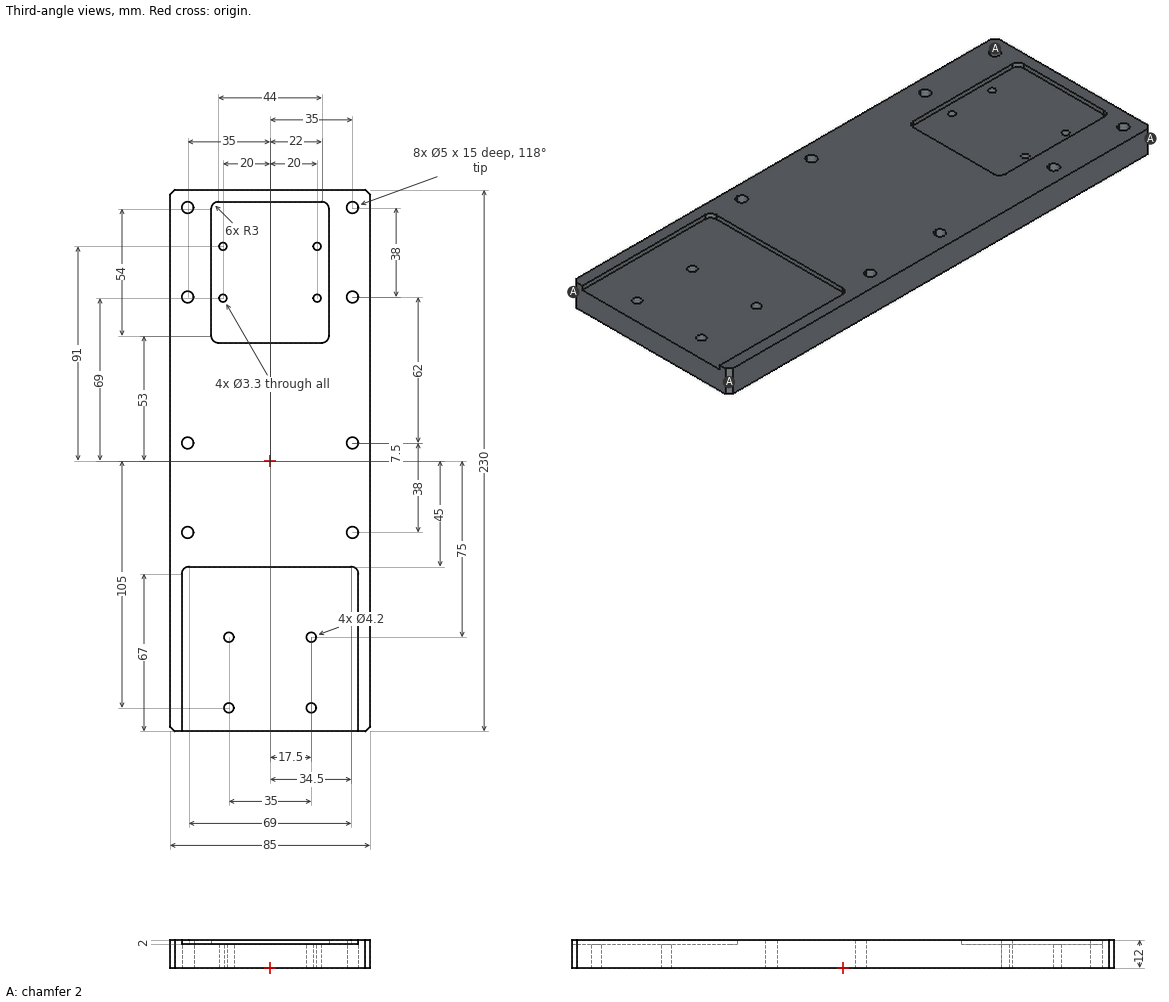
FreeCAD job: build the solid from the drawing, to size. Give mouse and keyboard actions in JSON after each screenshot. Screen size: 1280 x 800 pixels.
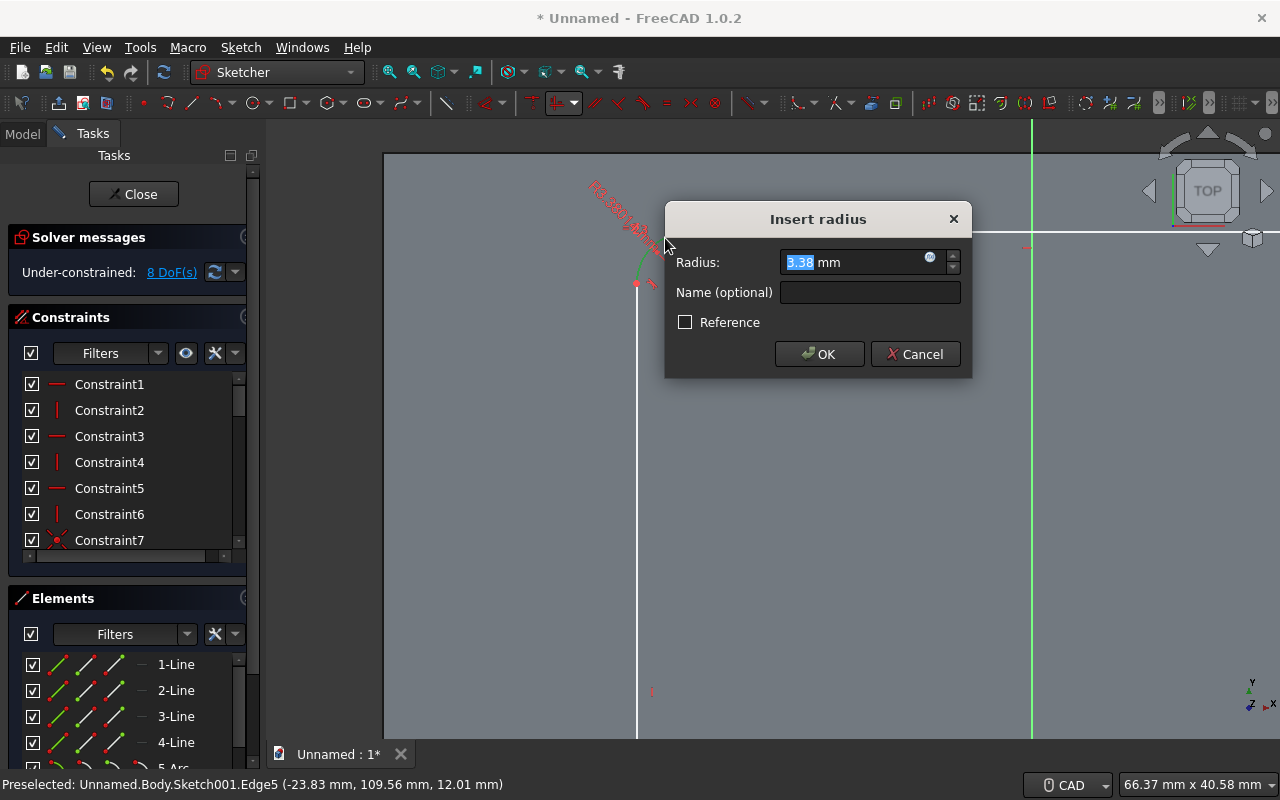
{"action": "type", "text": "3"}
{"action": "key", "text": "Return"}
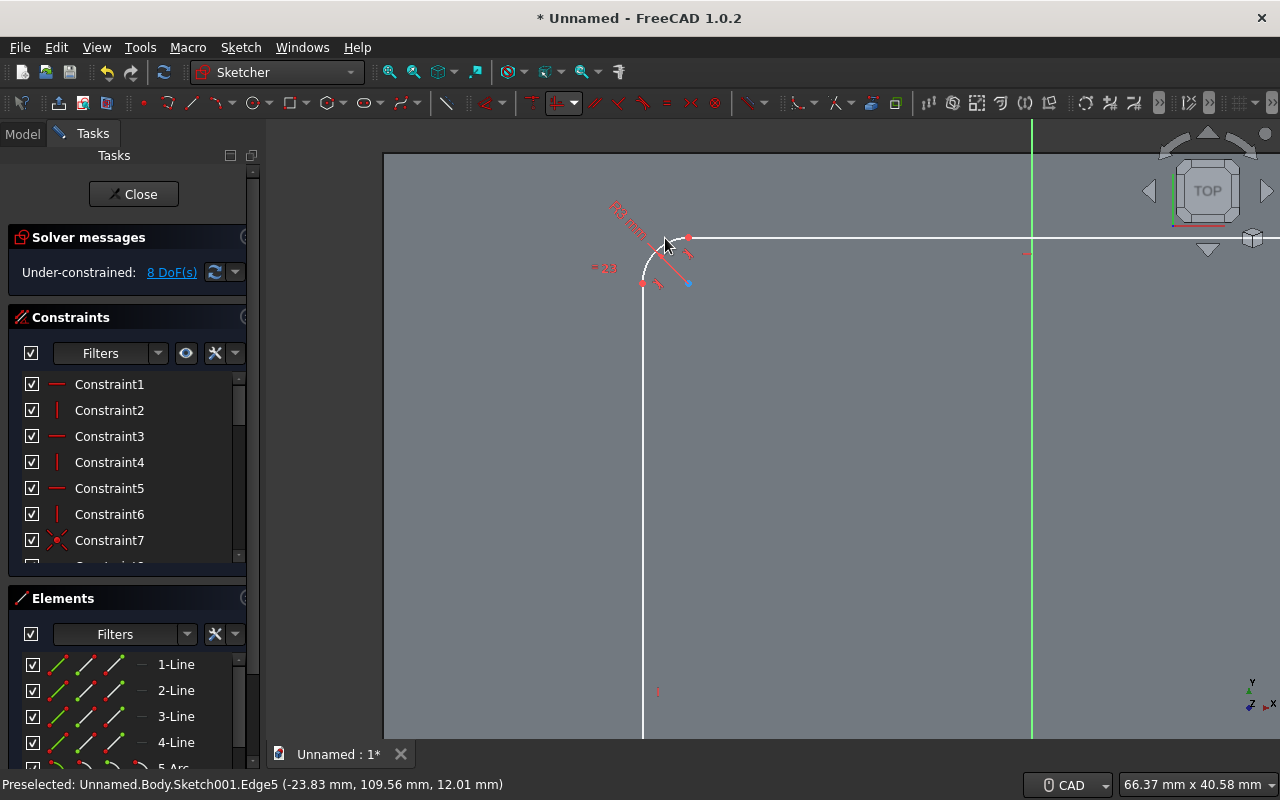
{"action": "scroll", "coordinate": [664, 240], "scroll_direction": "down", "scroll_amount": 11}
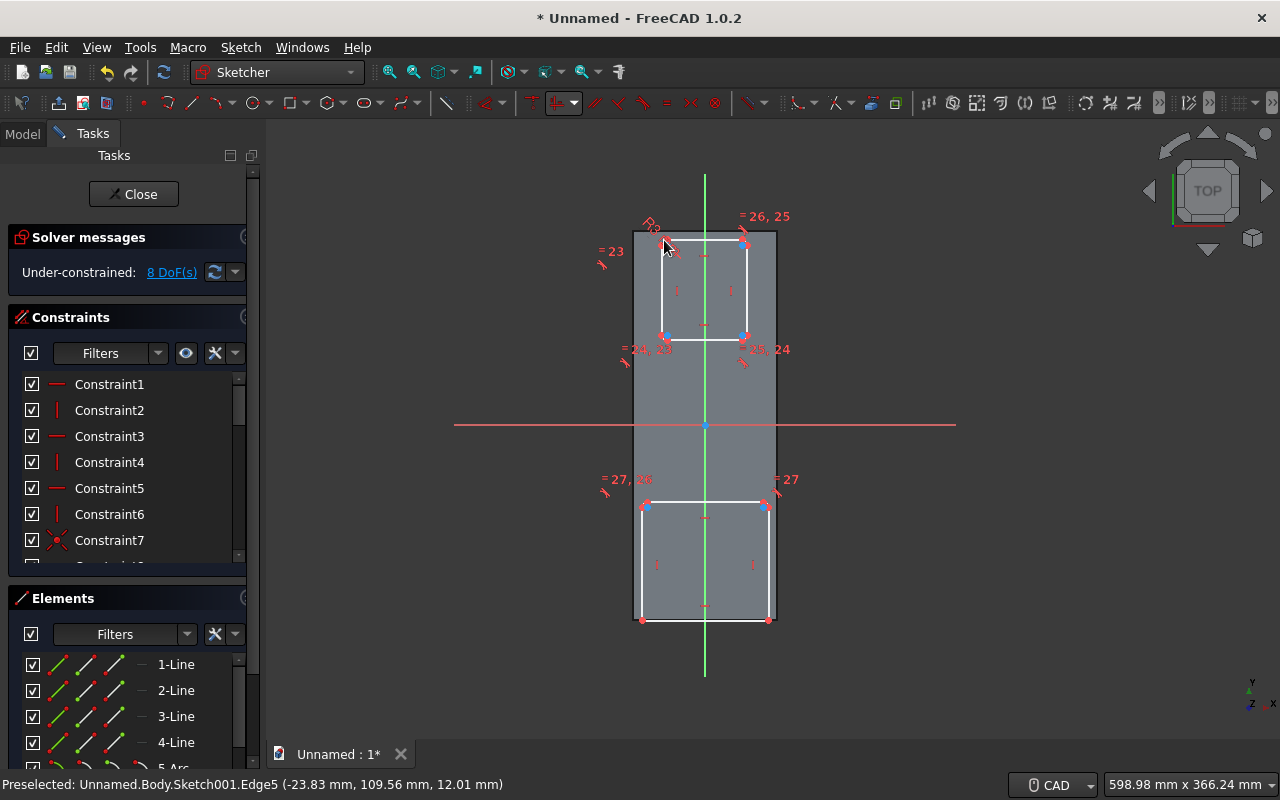
{"action": "left_click", "coordinate": [690, 240]}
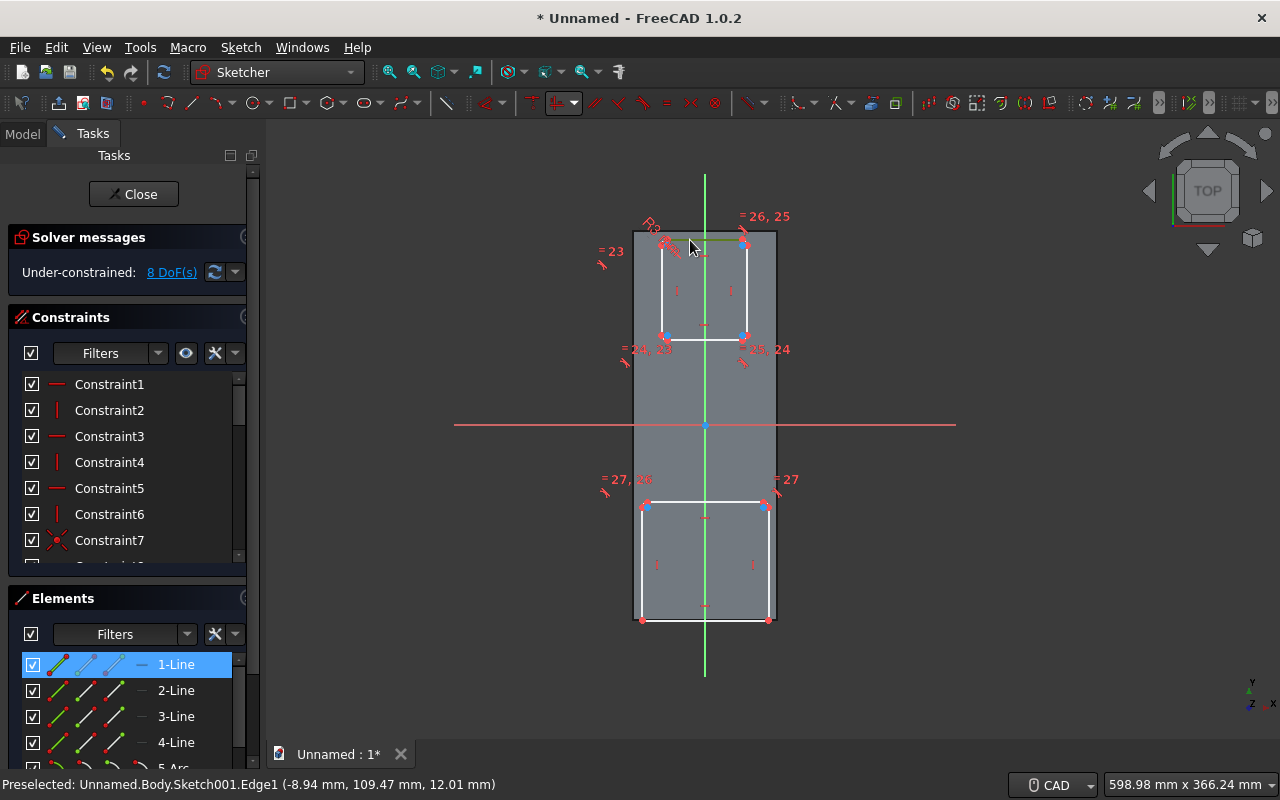
{"action": "key", "text": "l"}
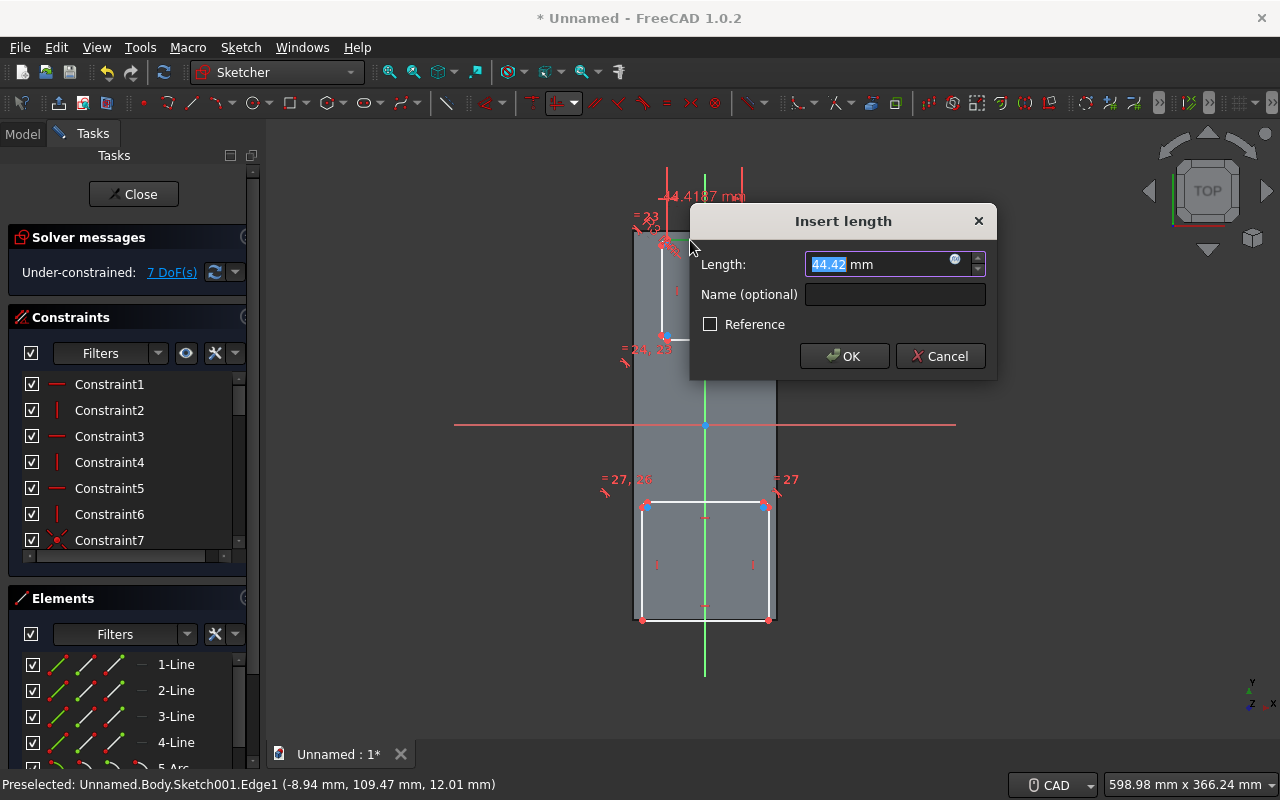
{"action": "type", "text": "44"}
{"action": "key", "text": "Return"}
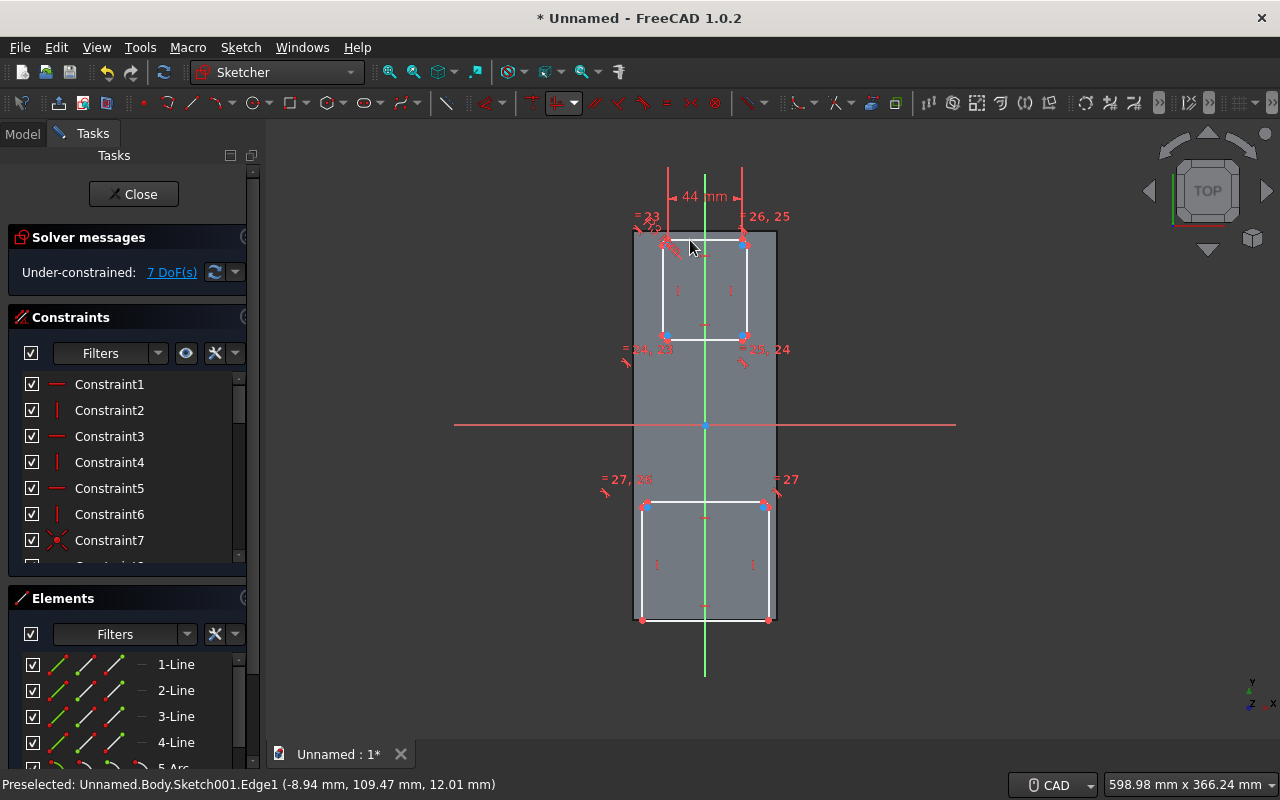
{"action": "left_click", "coordinate": [663, 272]}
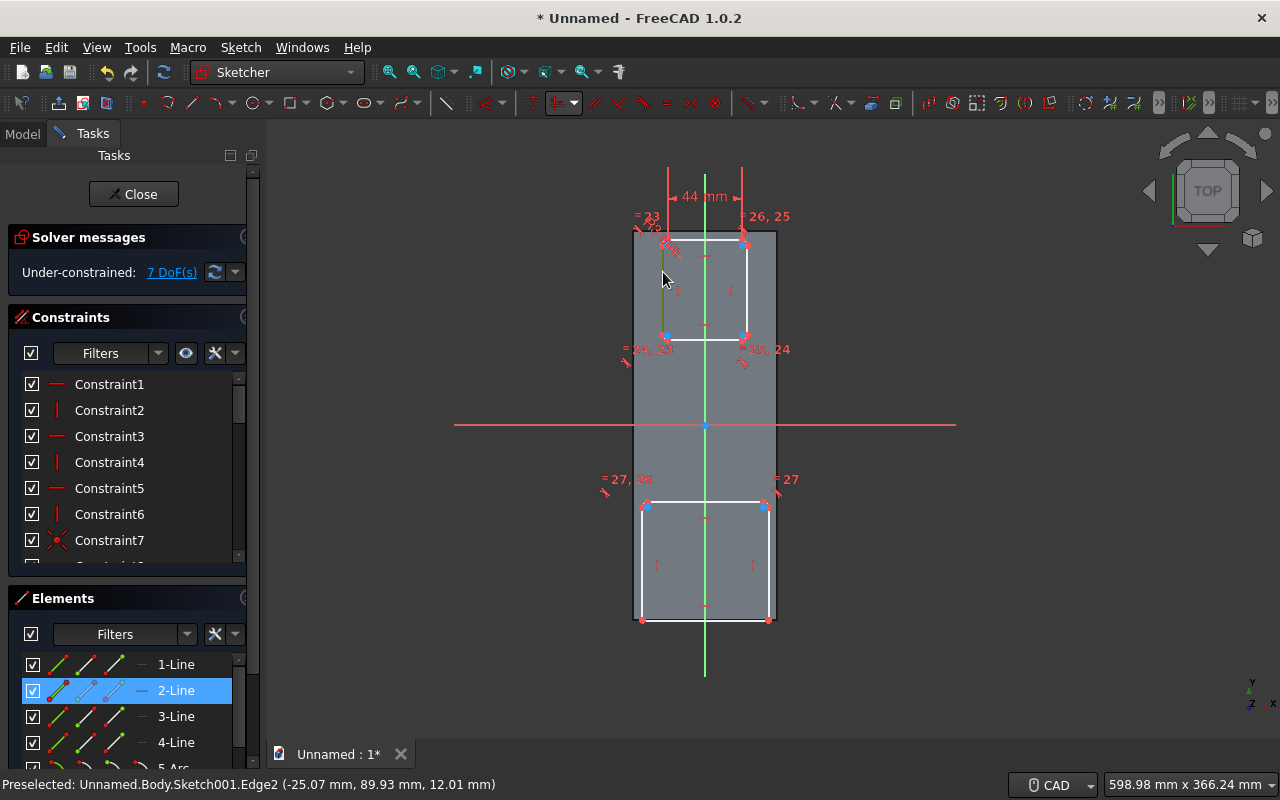
{"action": "key", "text": "i"}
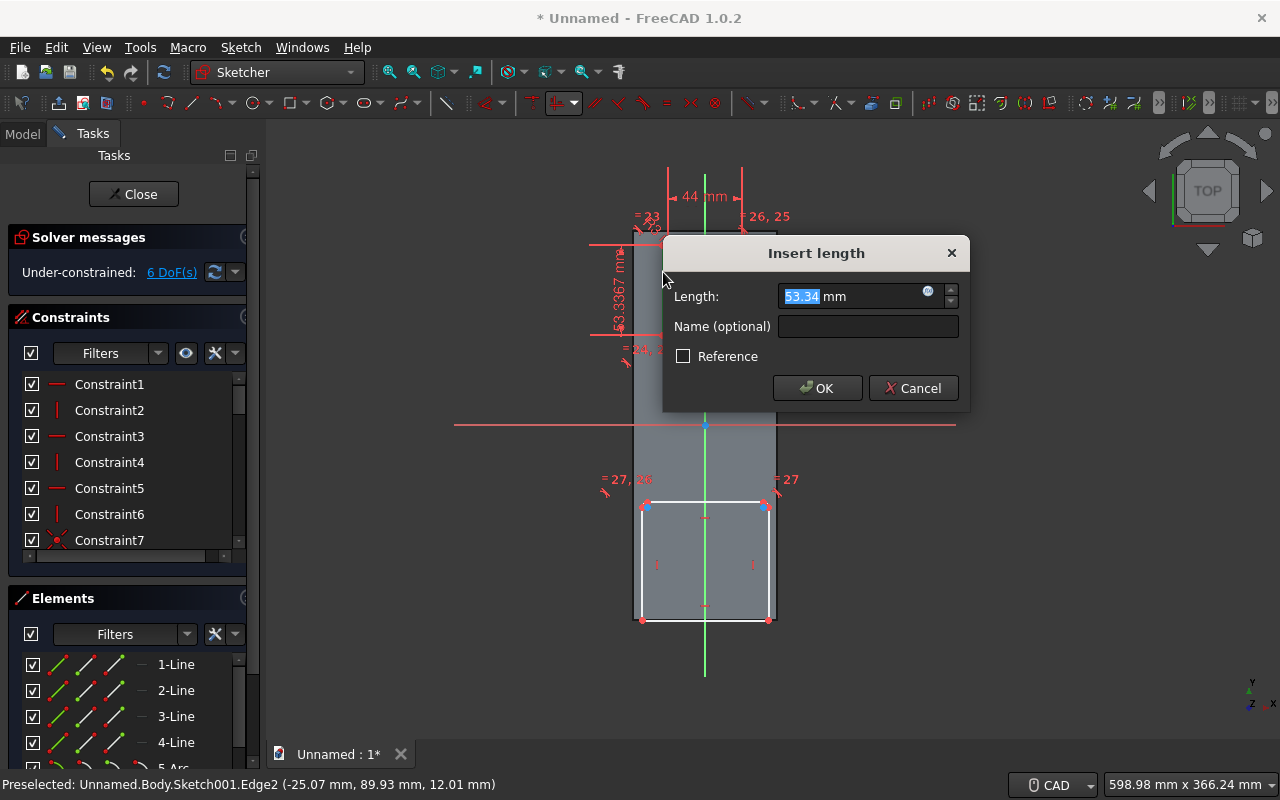
{"action": "type", "text": "54"}
{"action": "key", "text": "Return"}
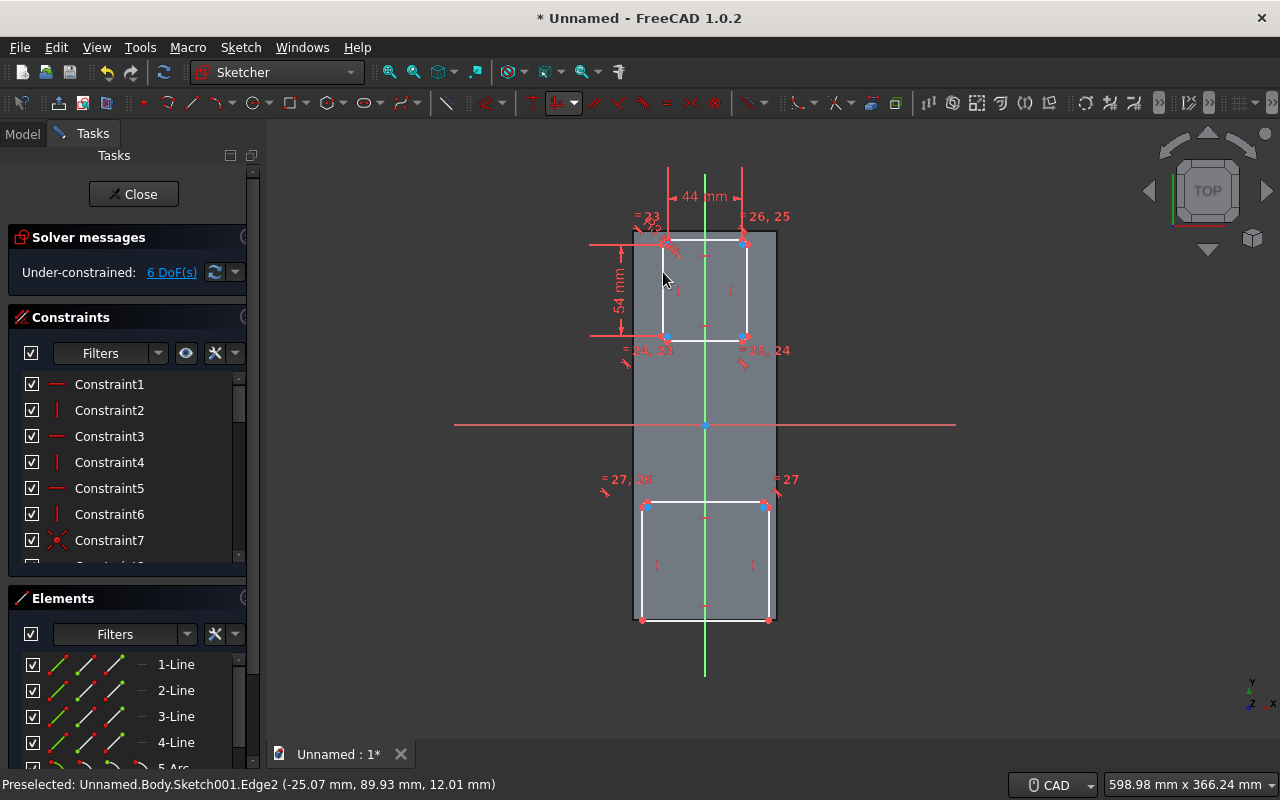
{"action": "left_click", "coordinate": [729, 502]}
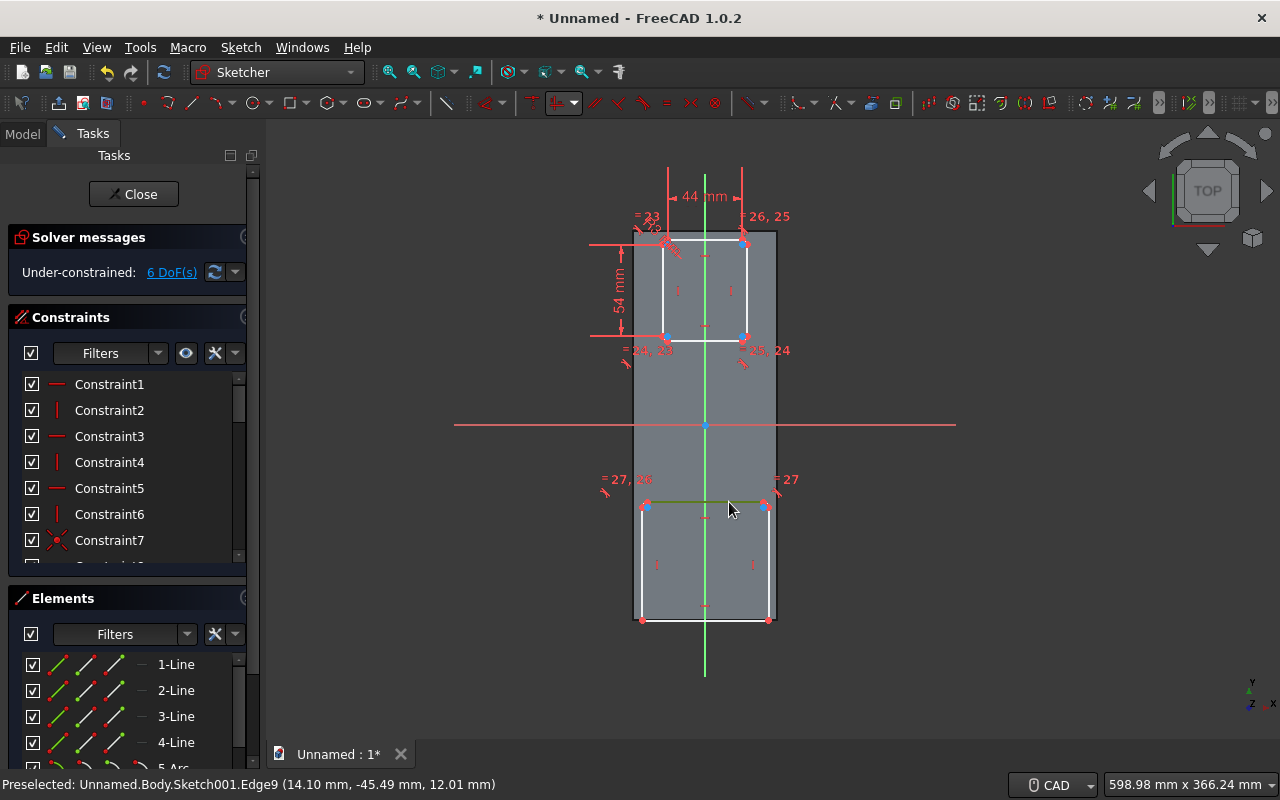
{"action": "key", "text": "l"}